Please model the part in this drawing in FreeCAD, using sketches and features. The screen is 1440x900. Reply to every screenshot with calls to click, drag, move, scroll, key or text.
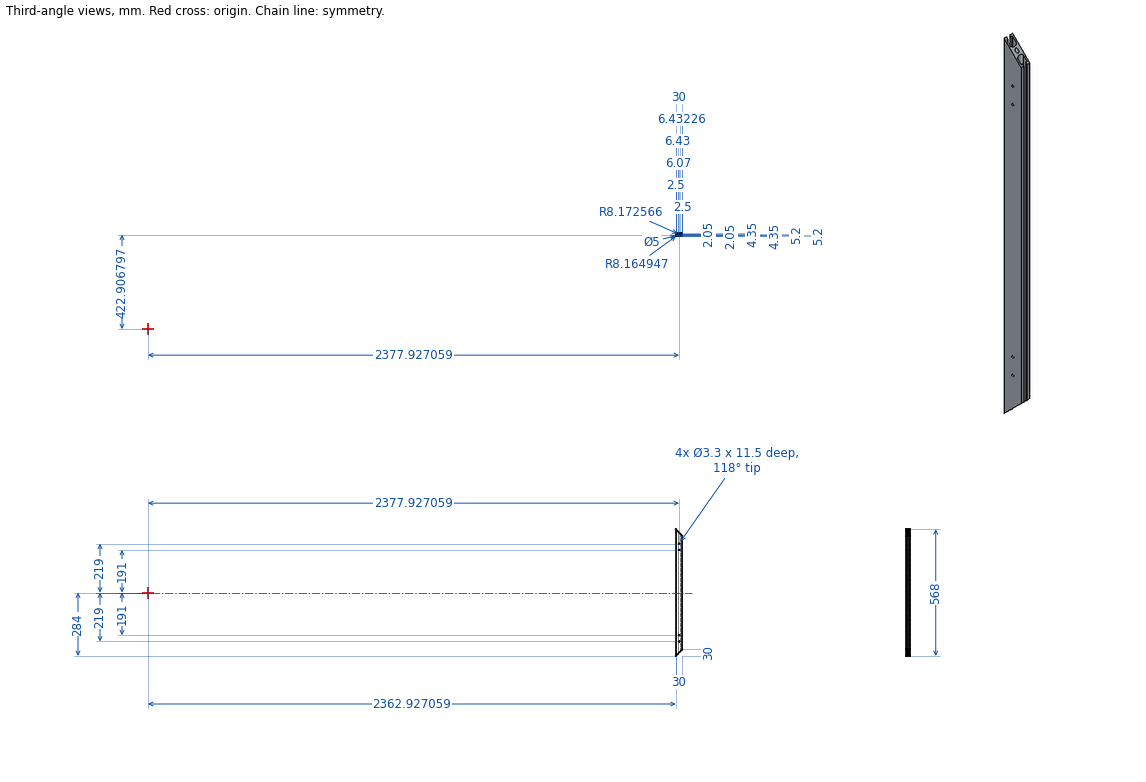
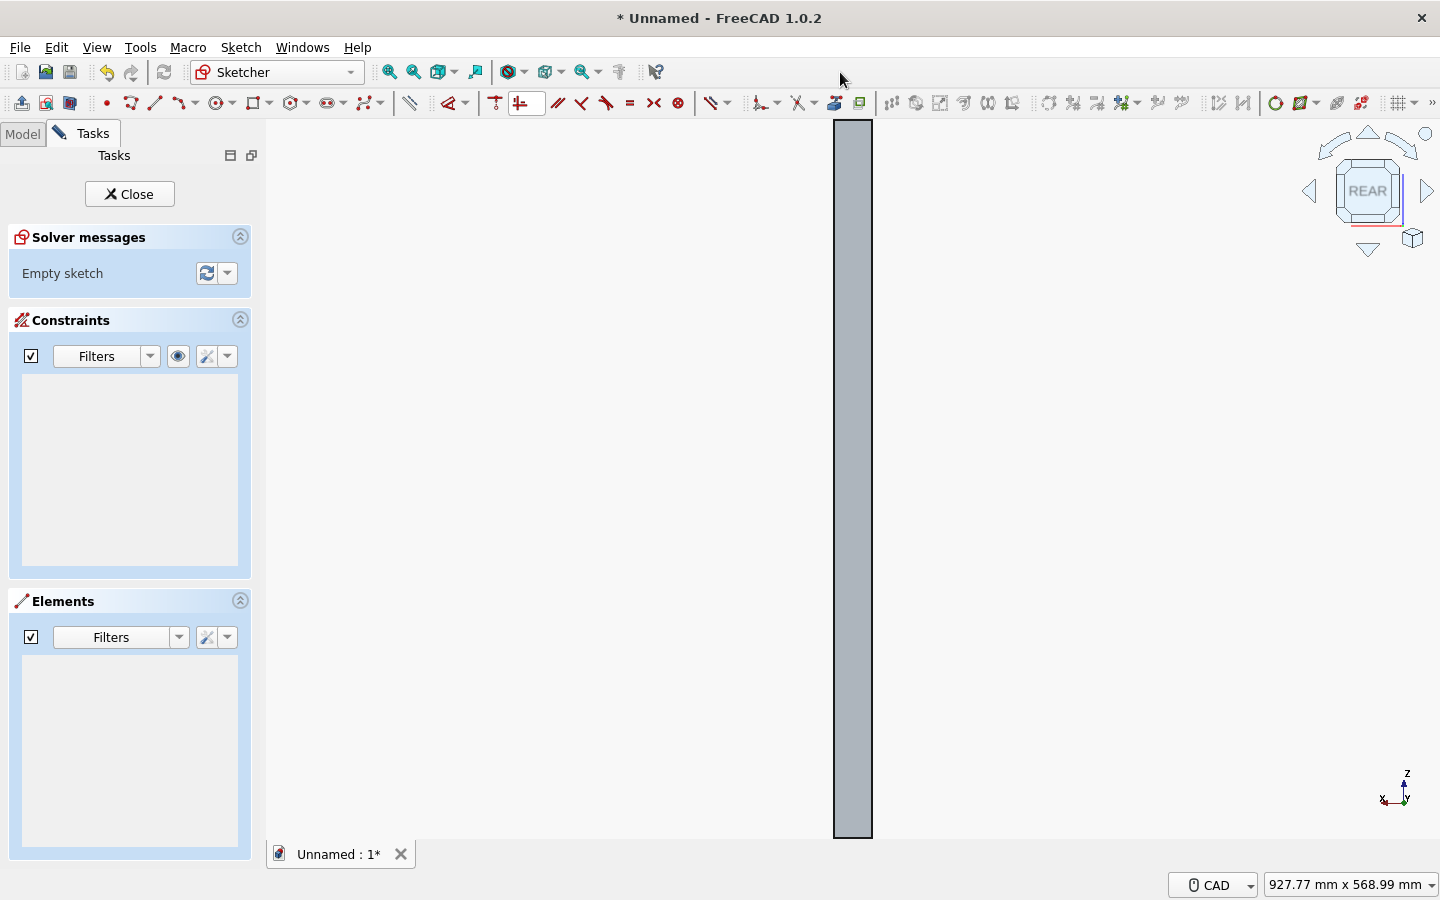
scroll(645, 479, down, 2)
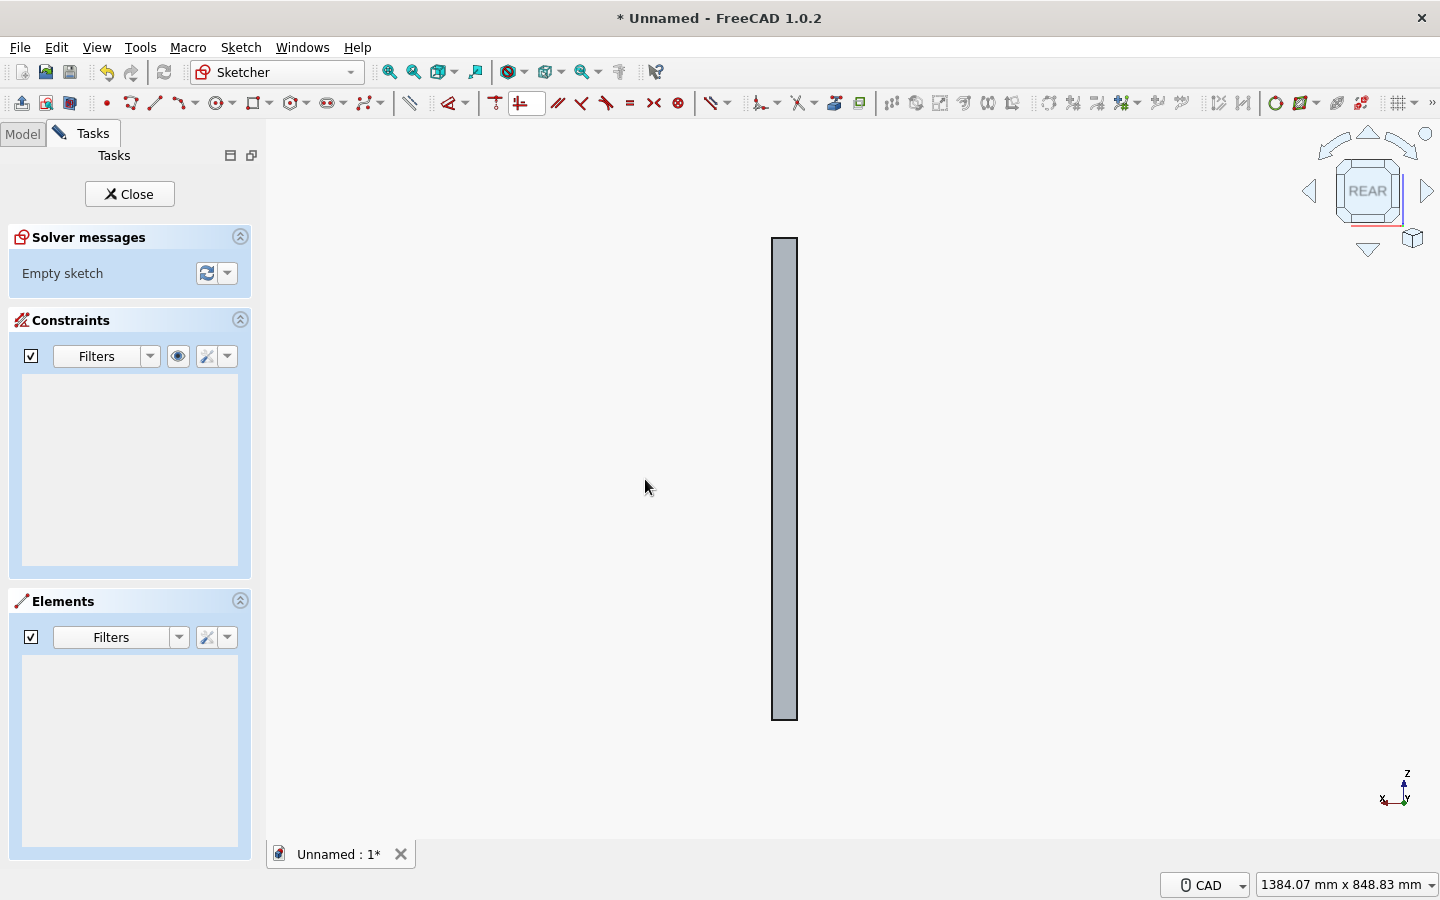
key(g)
key(m)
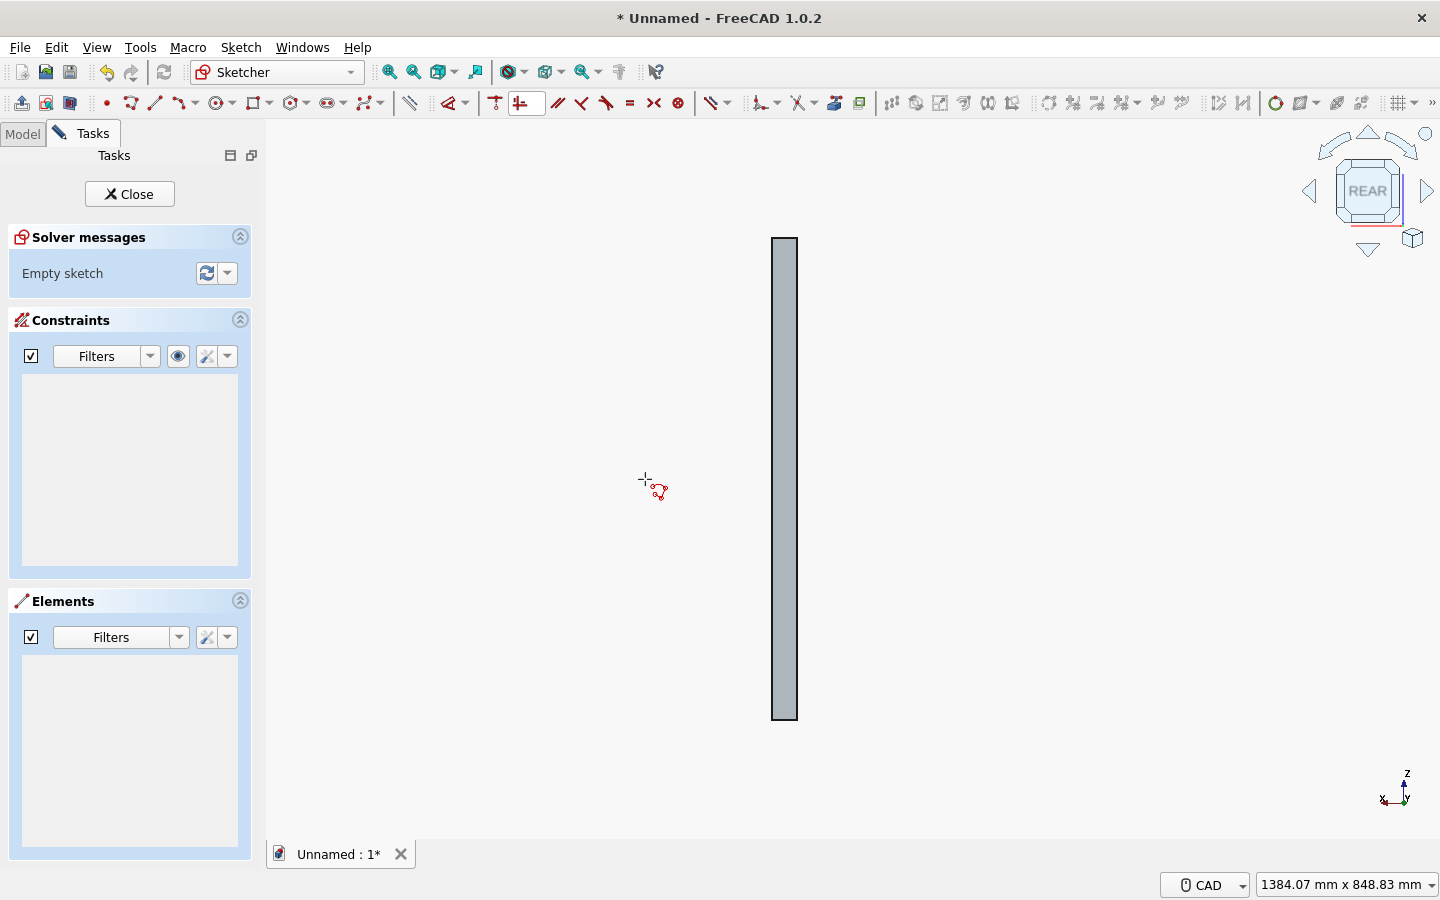
click(797, 720)
click(772, 695)
click(772, 720)
click(797, 721)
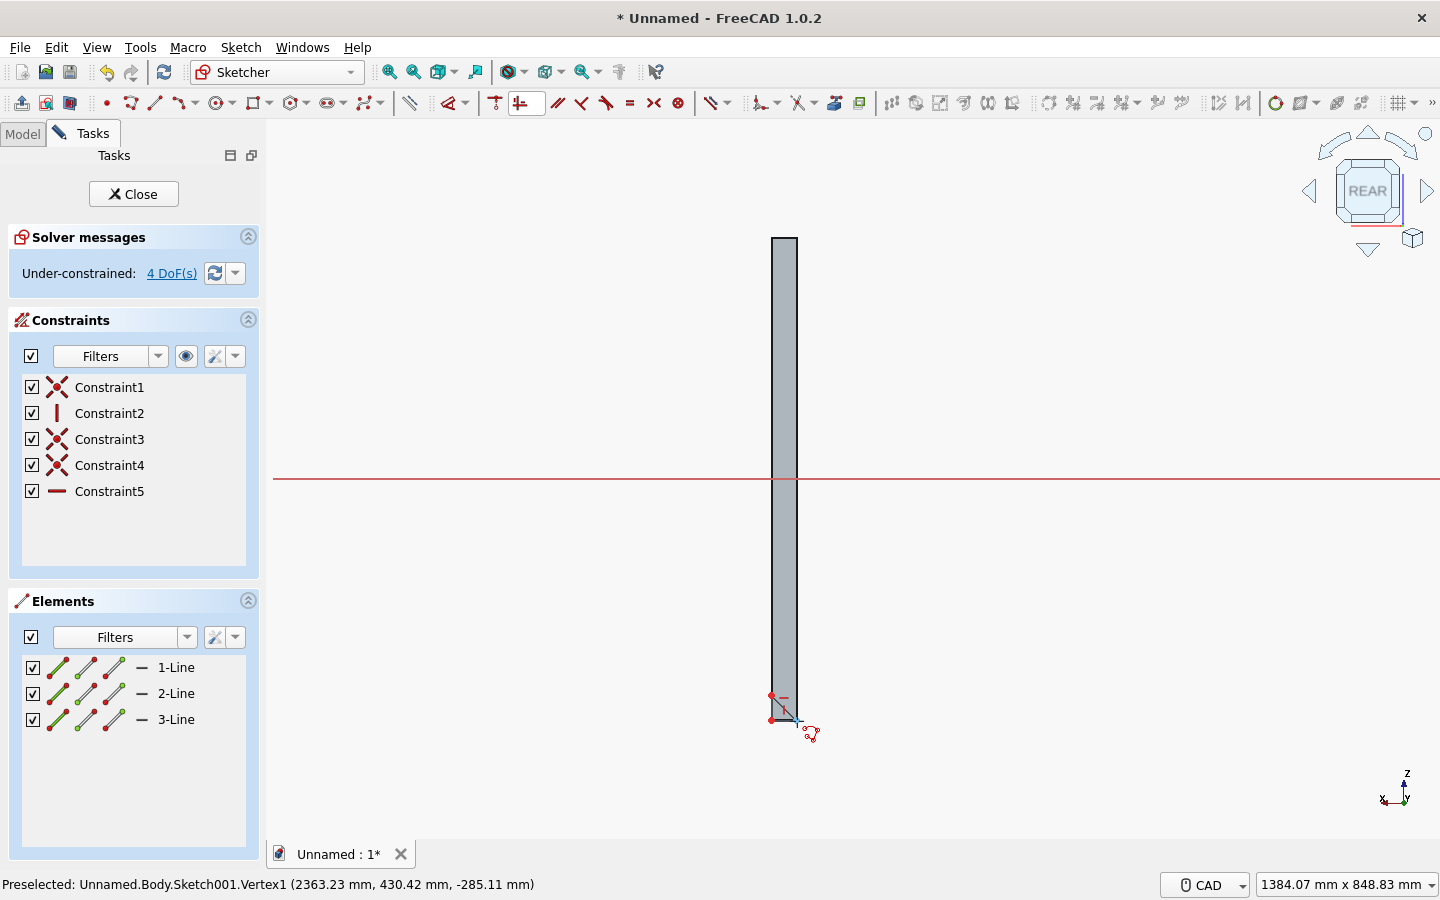
click(797, 238)
click(772, 238)
click(772, 264)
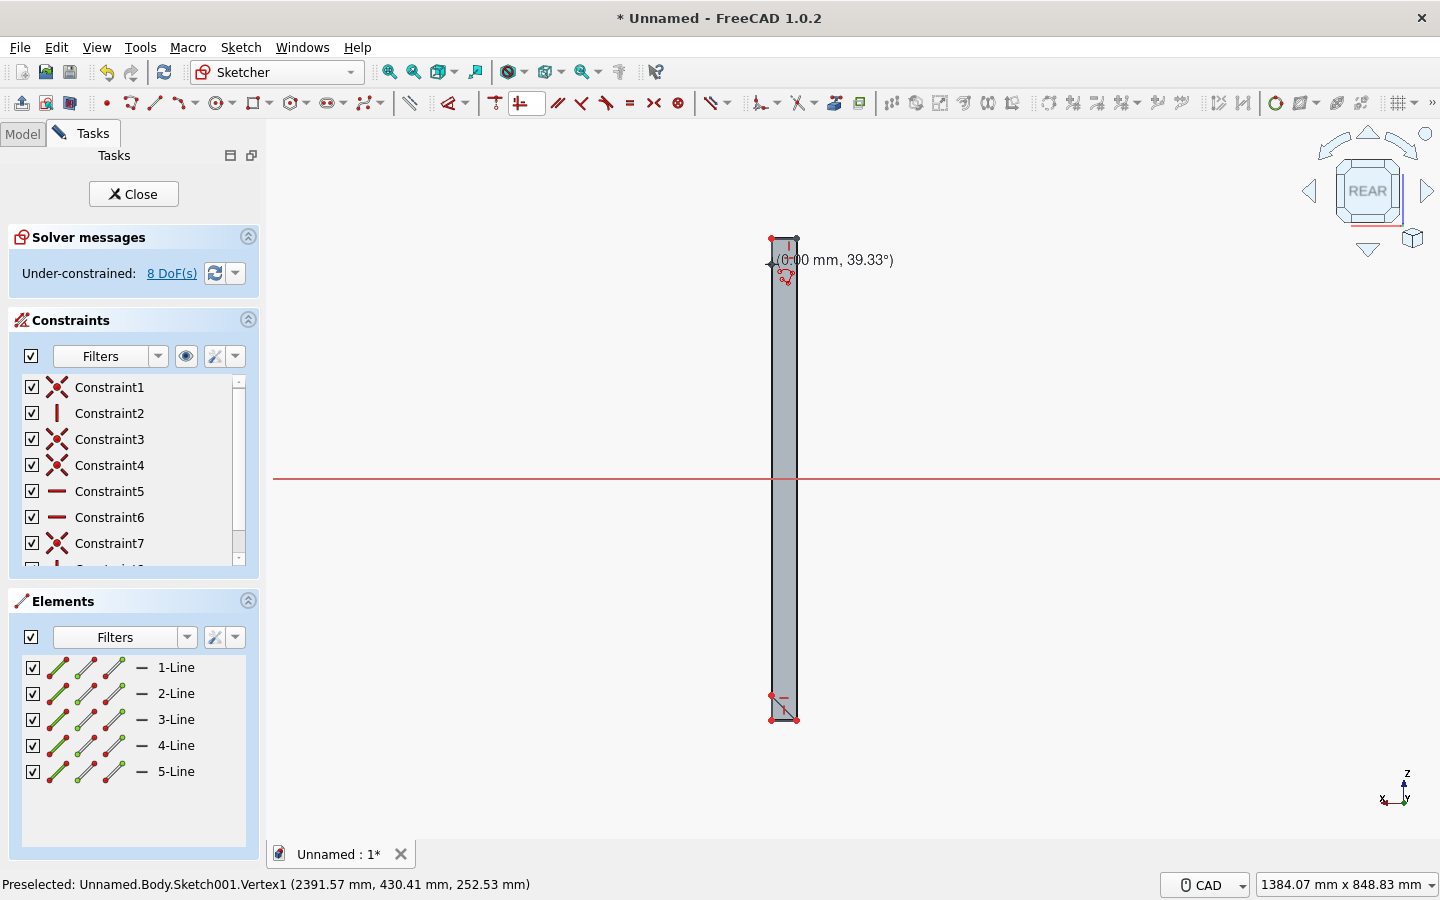
scroll(797, 238, up, 2)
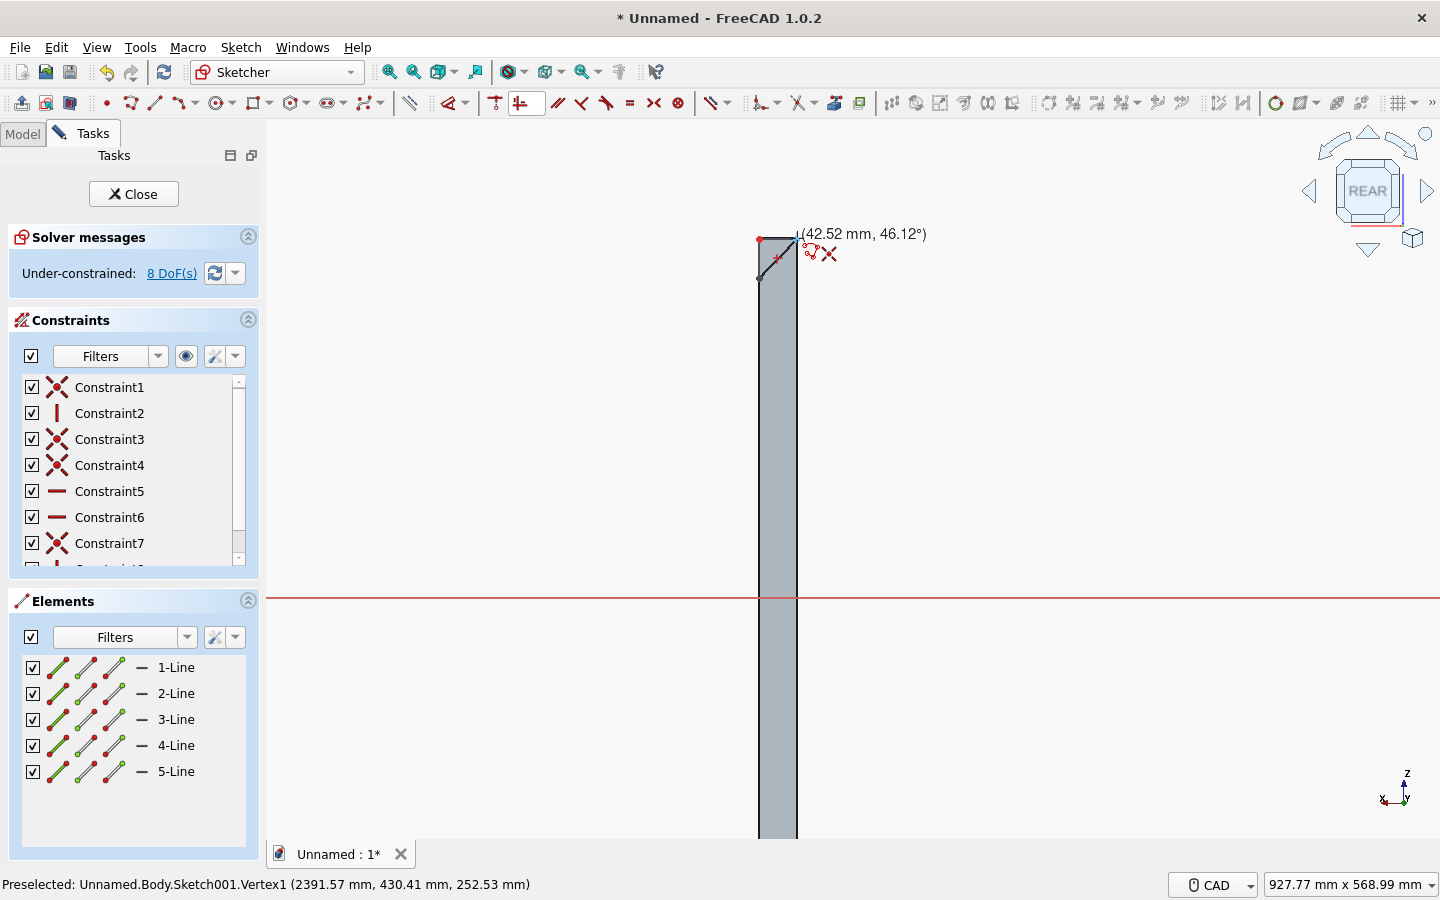
click(797, 239)
key(Escape)
key(Escape)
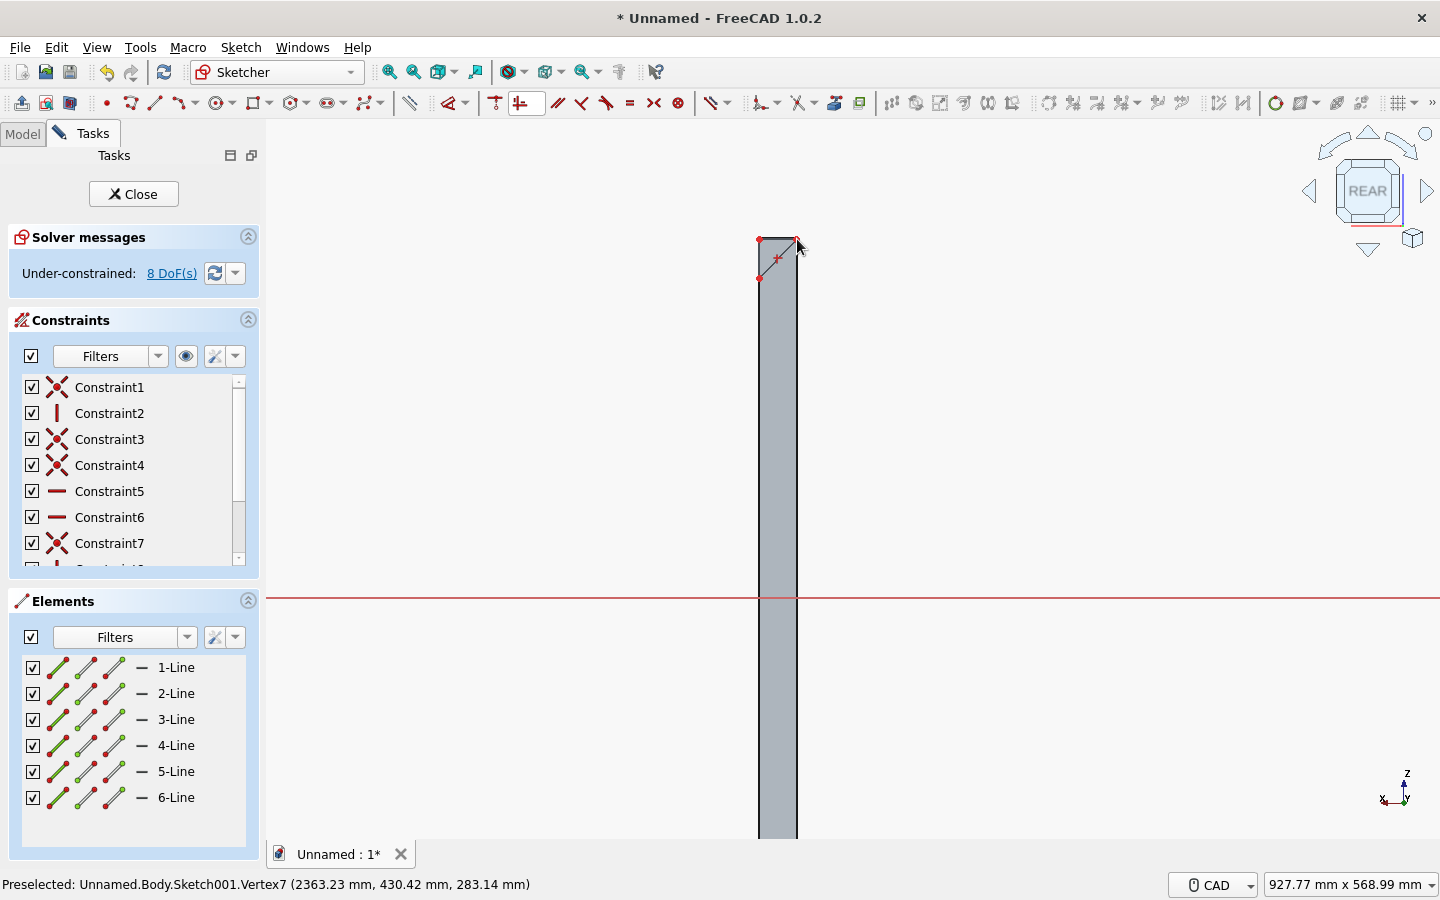
scroll(797, 238, down, 2)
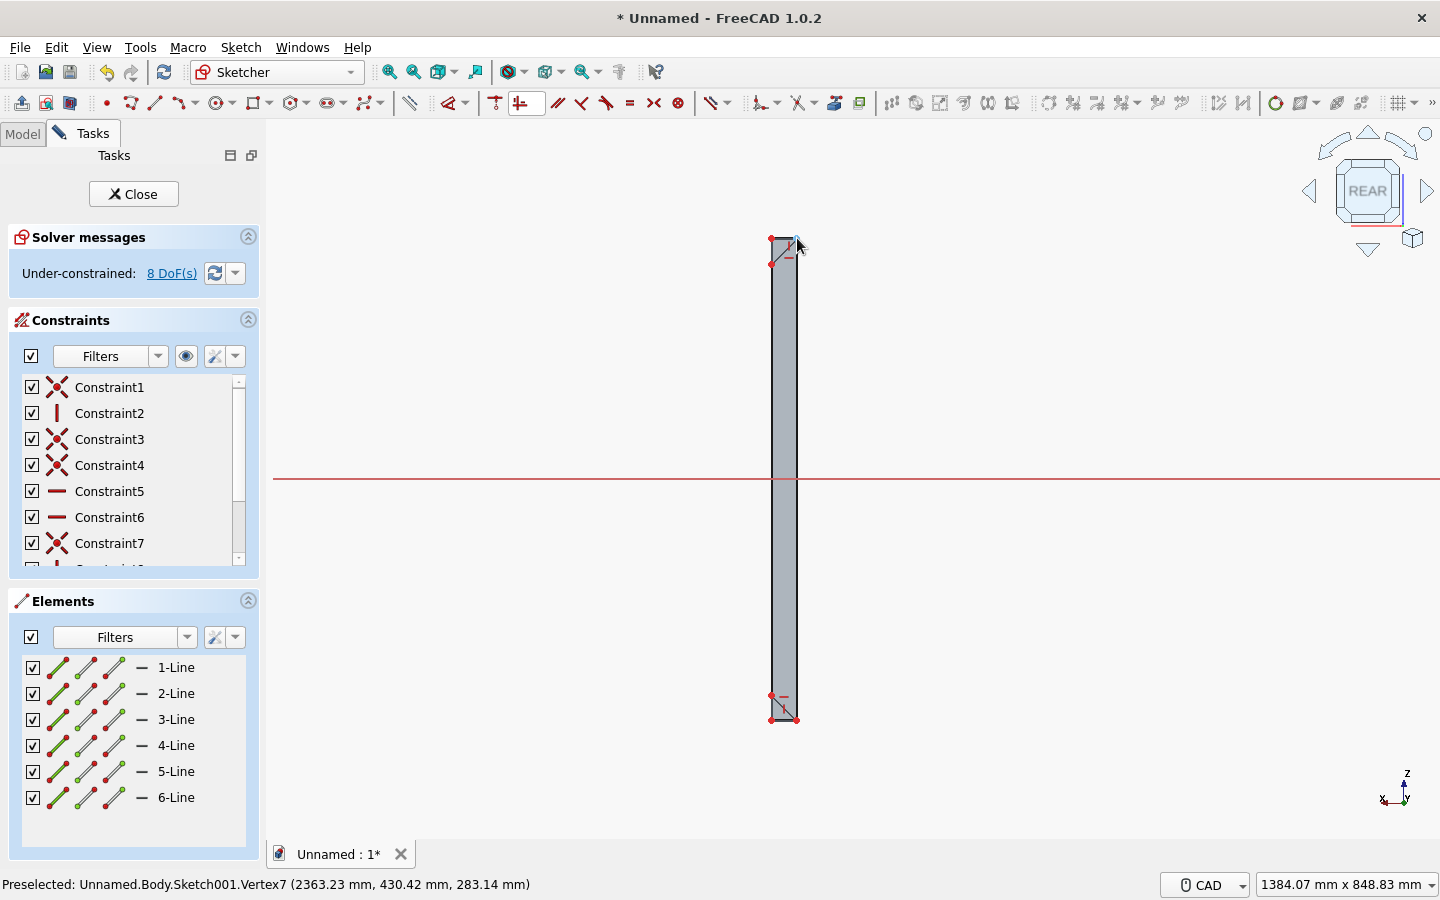
click(797, 721)